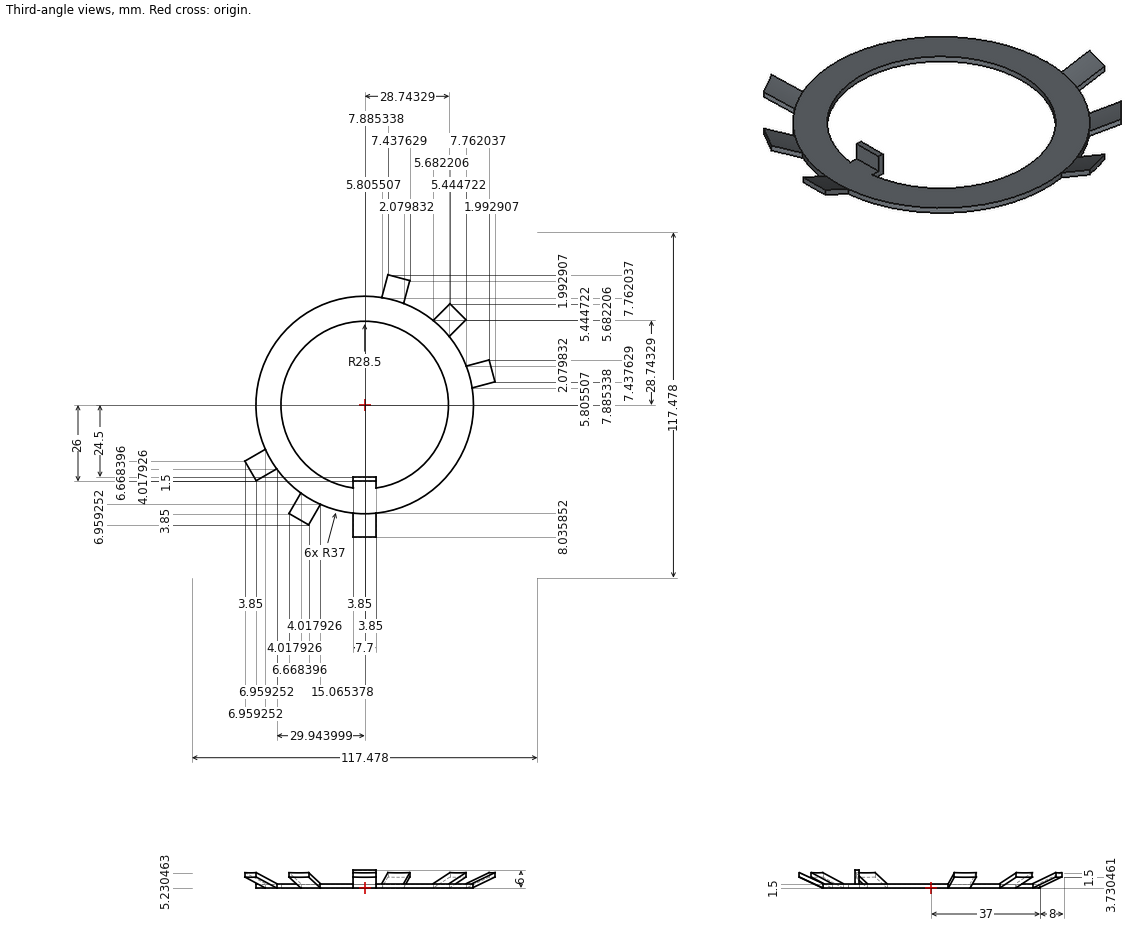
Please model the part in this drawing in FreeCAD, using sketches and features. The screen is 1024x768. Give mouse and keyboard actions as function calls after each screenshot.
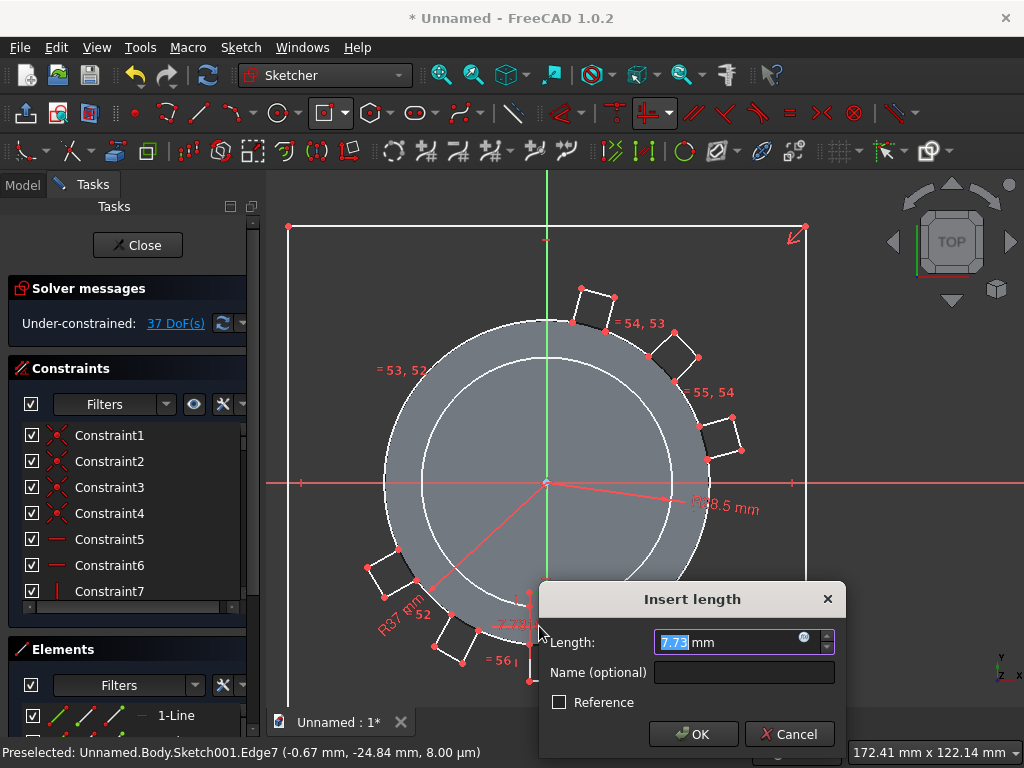
text(7.7)
key(Return)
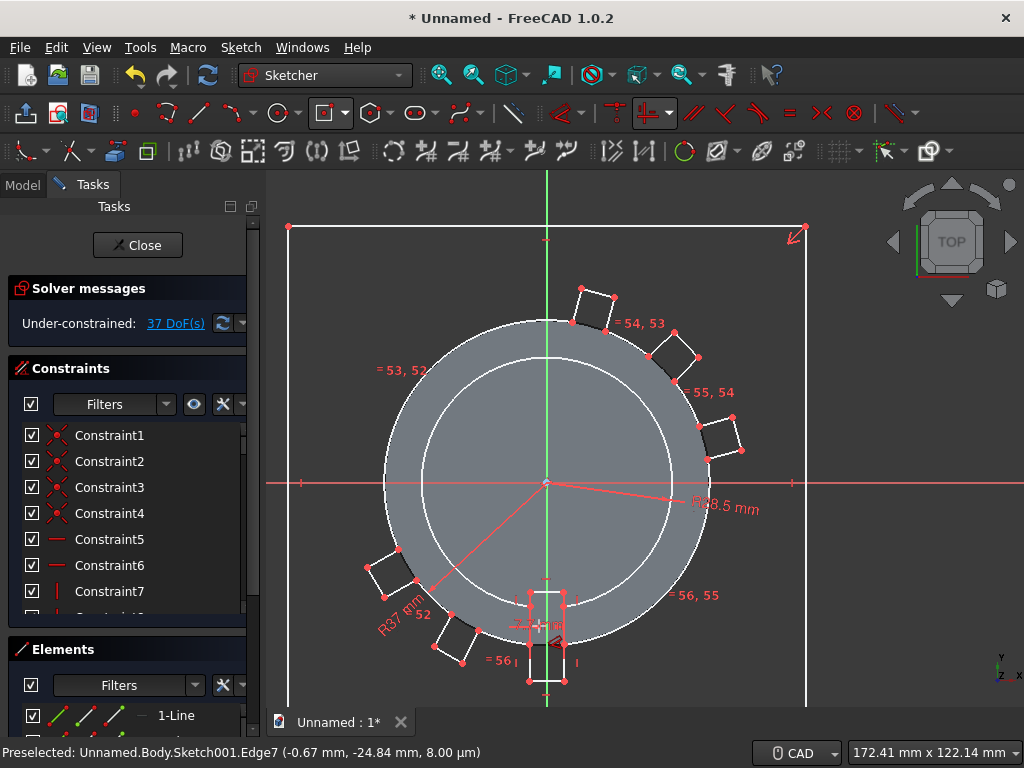
scroll(637, 348, down, 2)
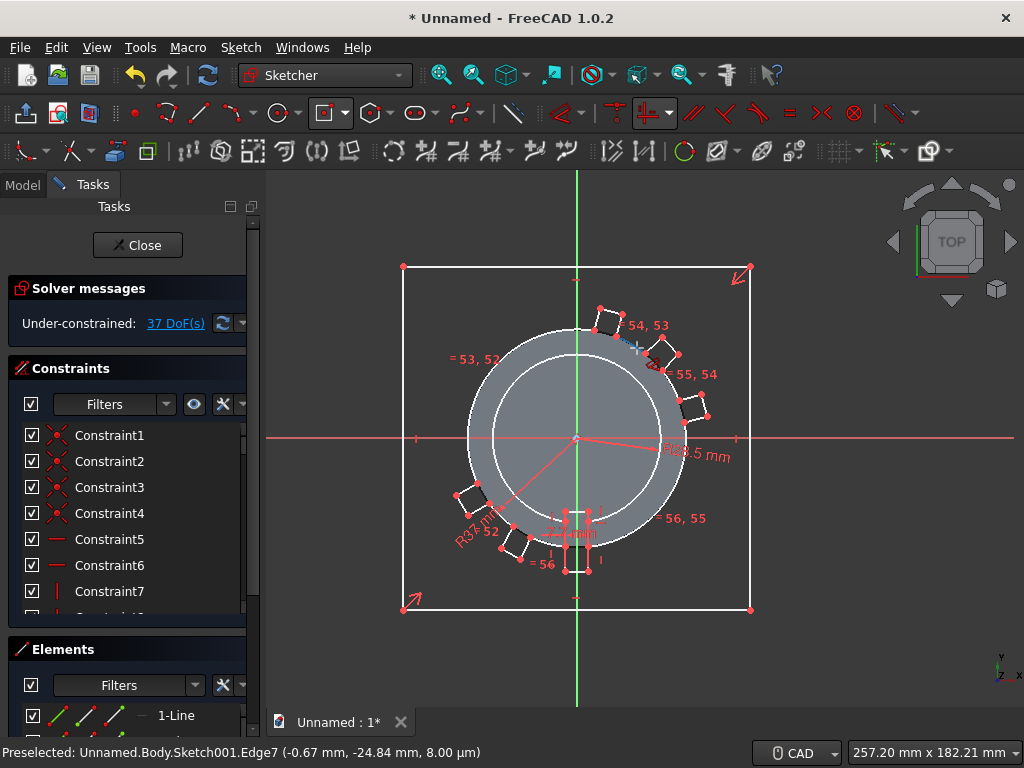
scroll(579, 572, up, 3)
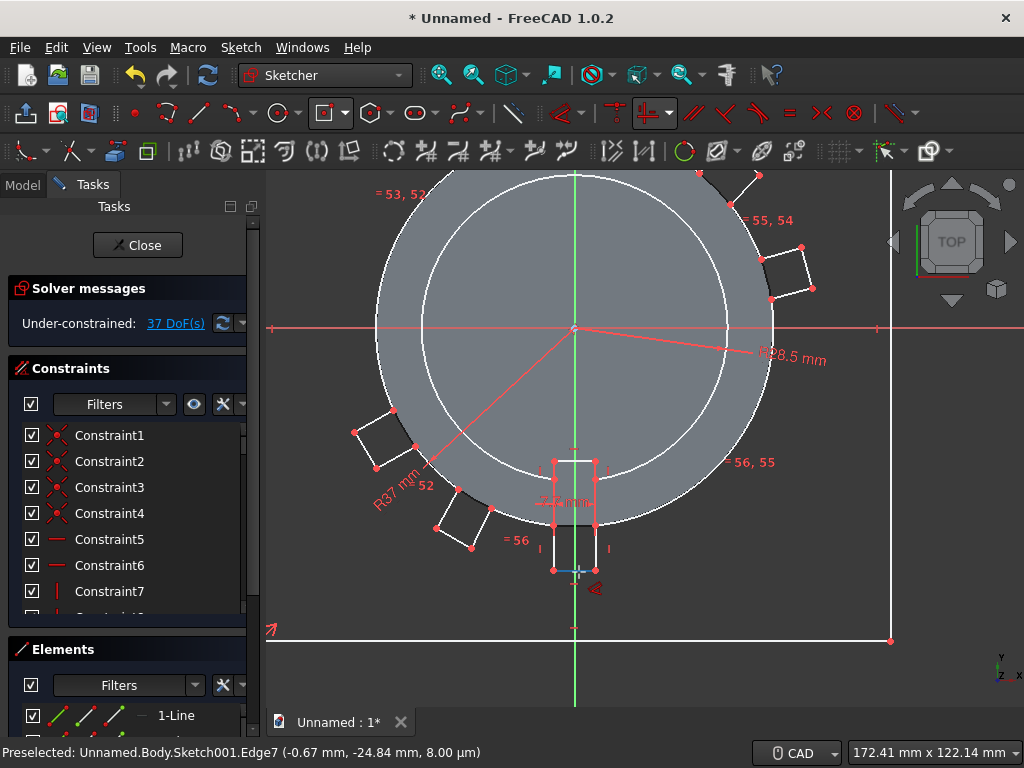
click(579, 571)
click(560, 605)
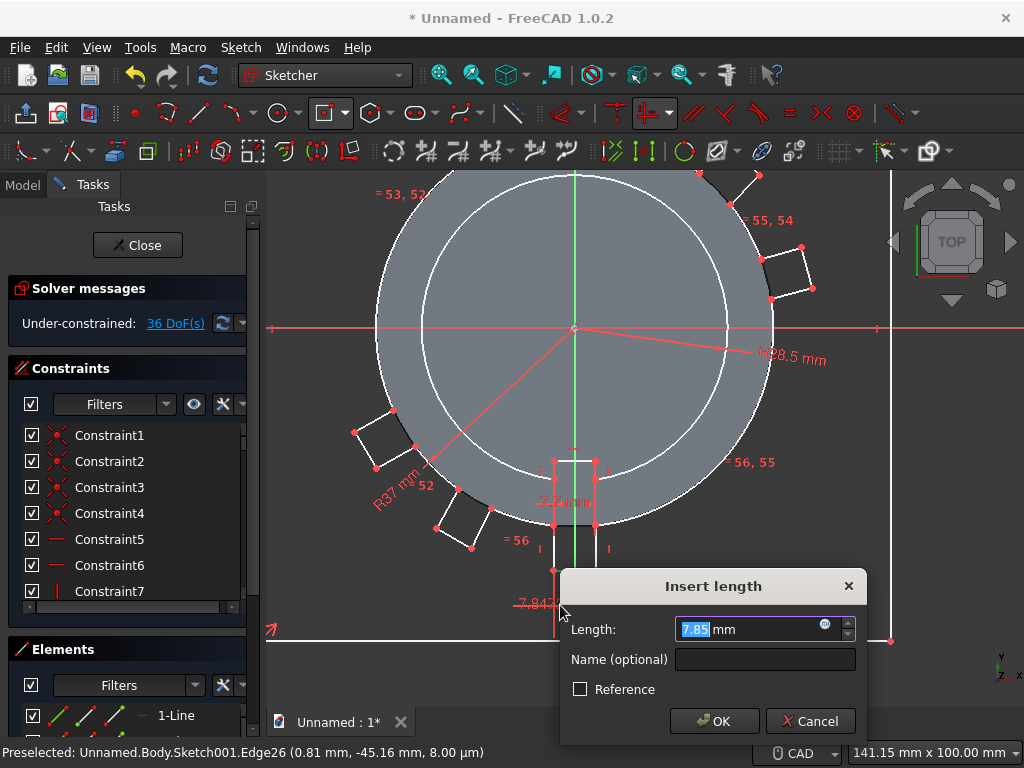
text(7.7)
key(Return)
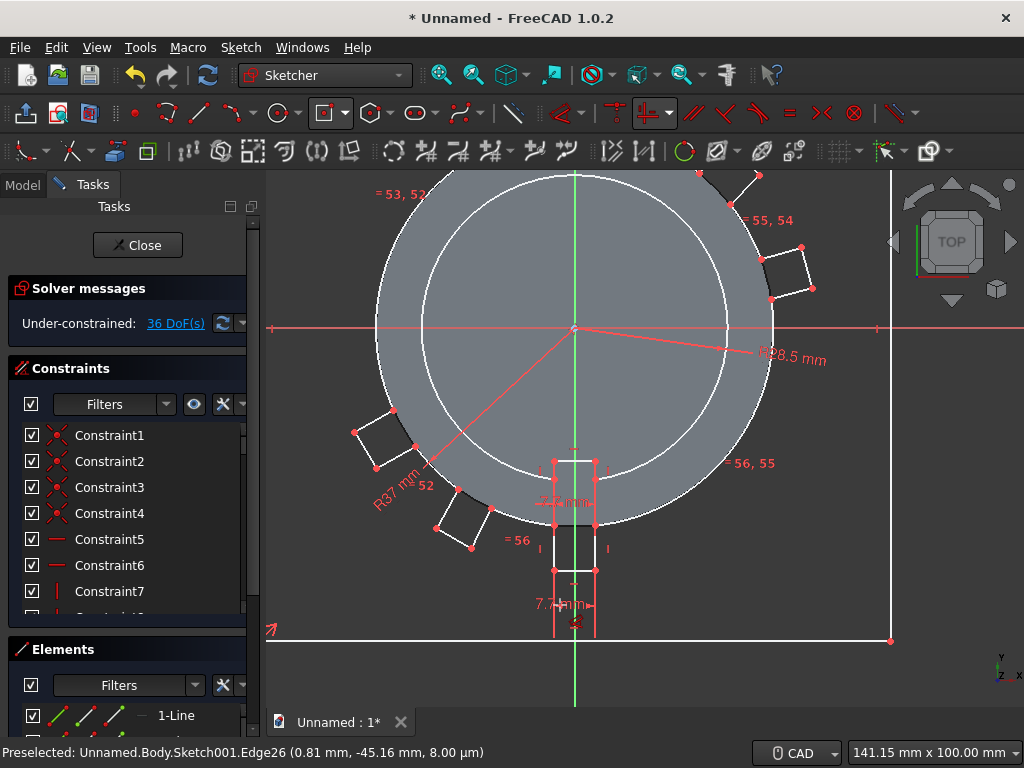
scroll(554, 480, up, 4)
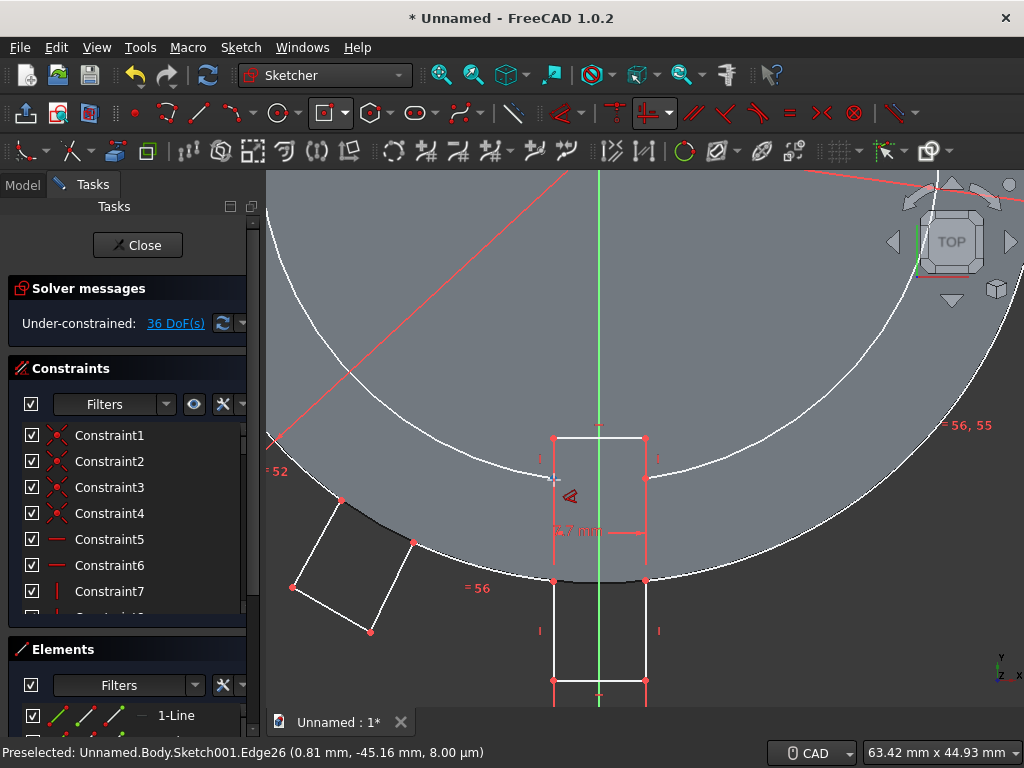
click(554, 479)
click(577, 561)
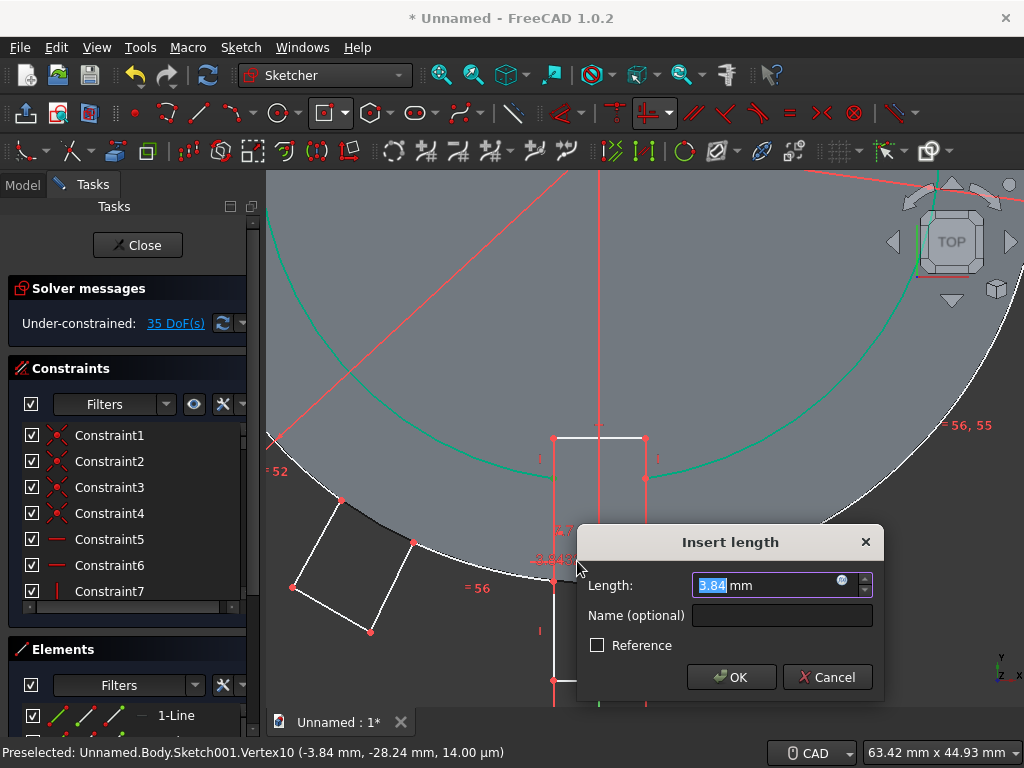
text(3.85)
key(Return)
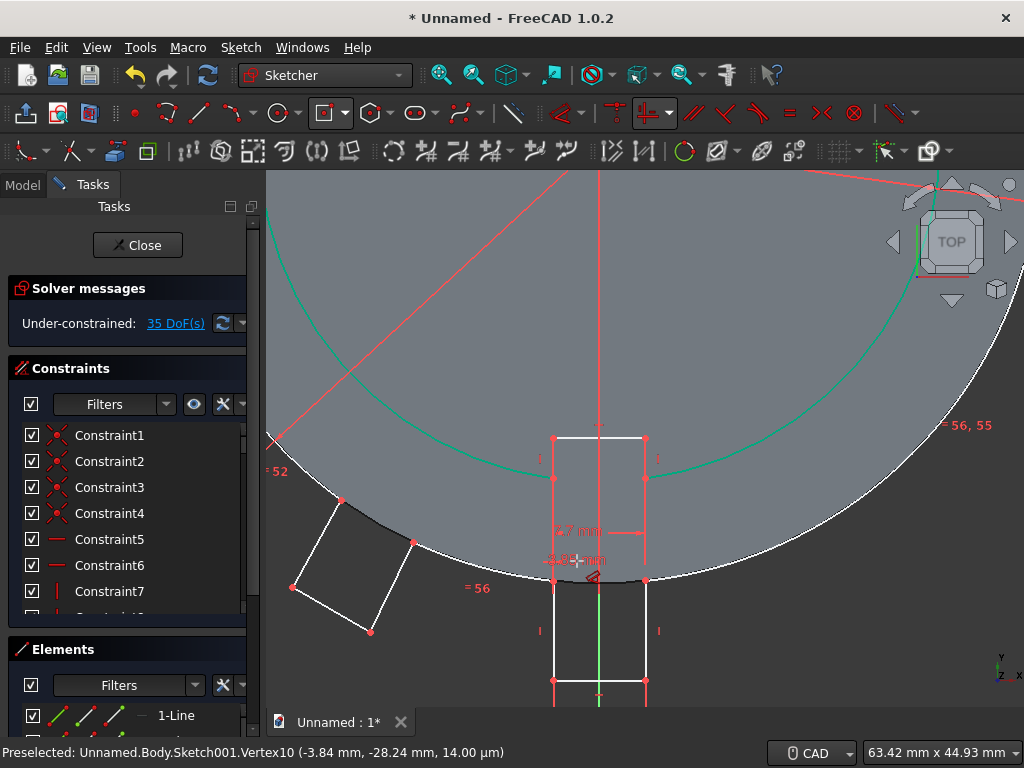
scroll(569, 536, down, 7)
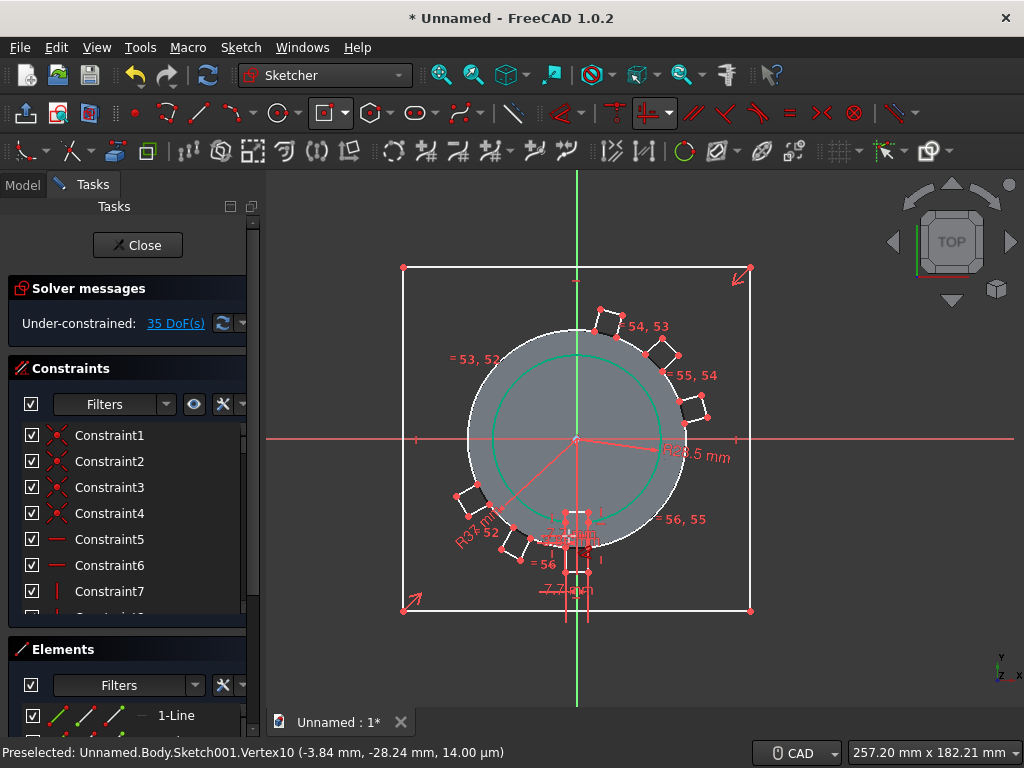
click(565, 512)
click(531, 476)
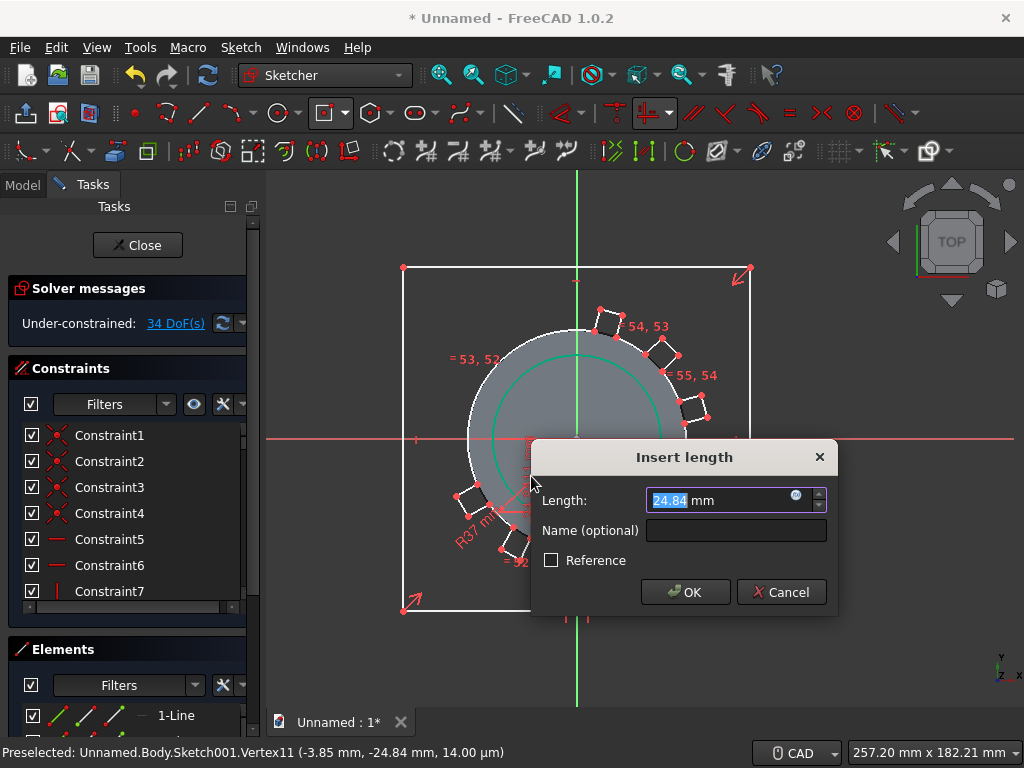
text(24.5)
key(Return)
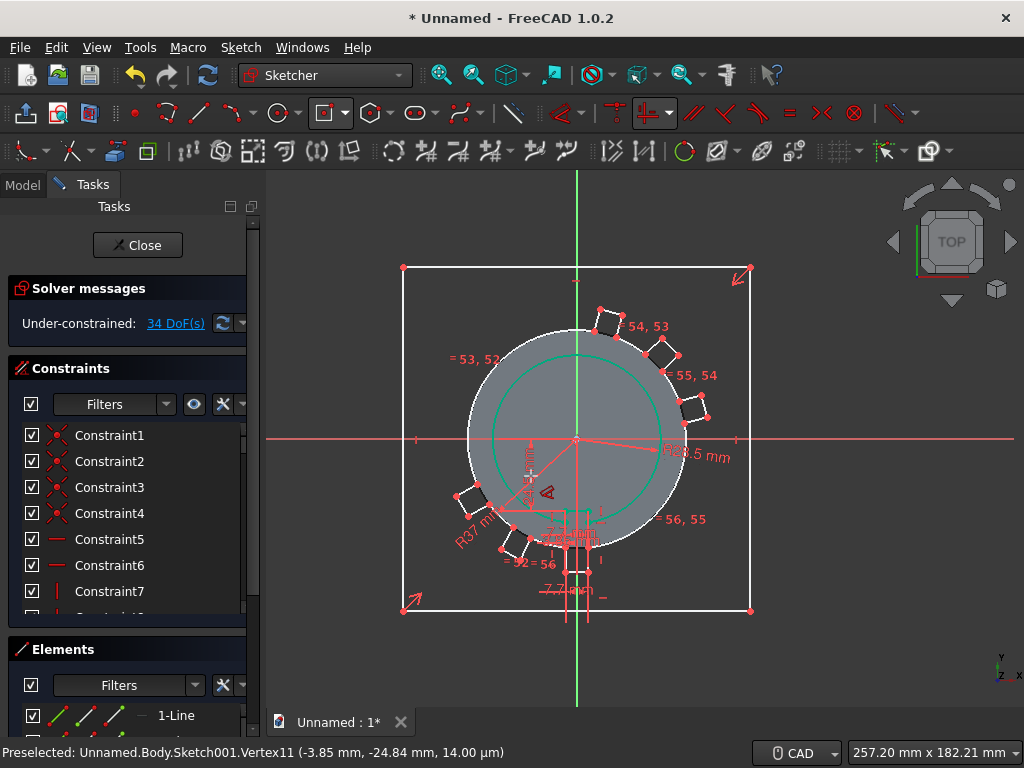
scroll(588, 548, up, 7)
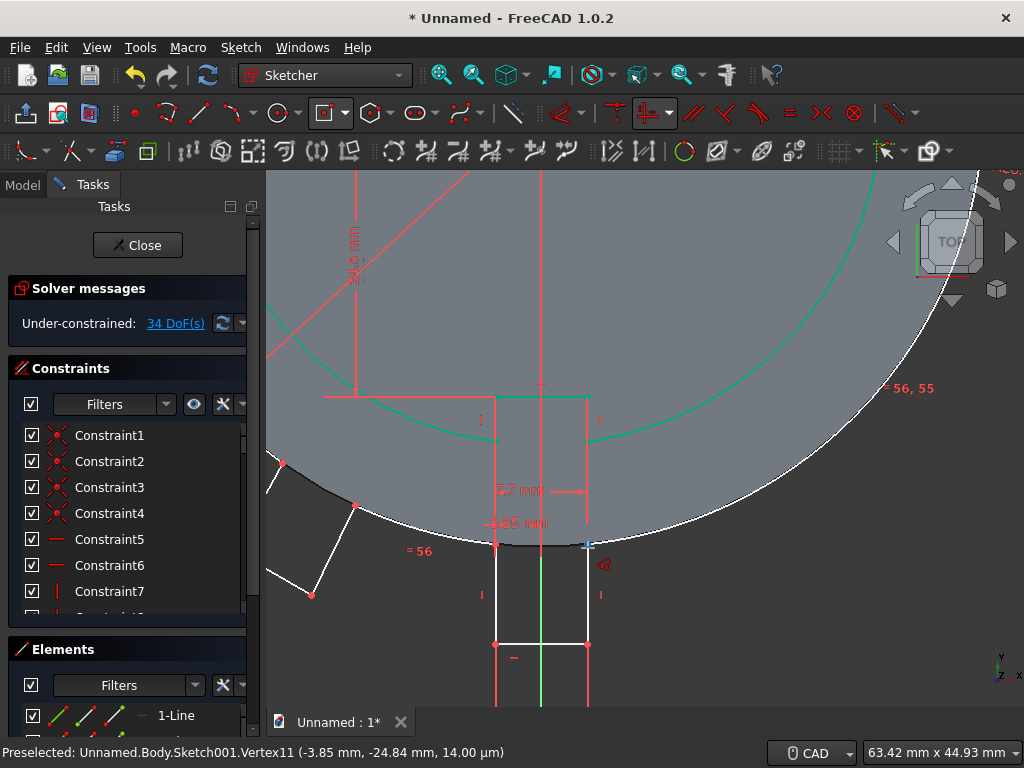
click(588, 544)
click(564, 578)